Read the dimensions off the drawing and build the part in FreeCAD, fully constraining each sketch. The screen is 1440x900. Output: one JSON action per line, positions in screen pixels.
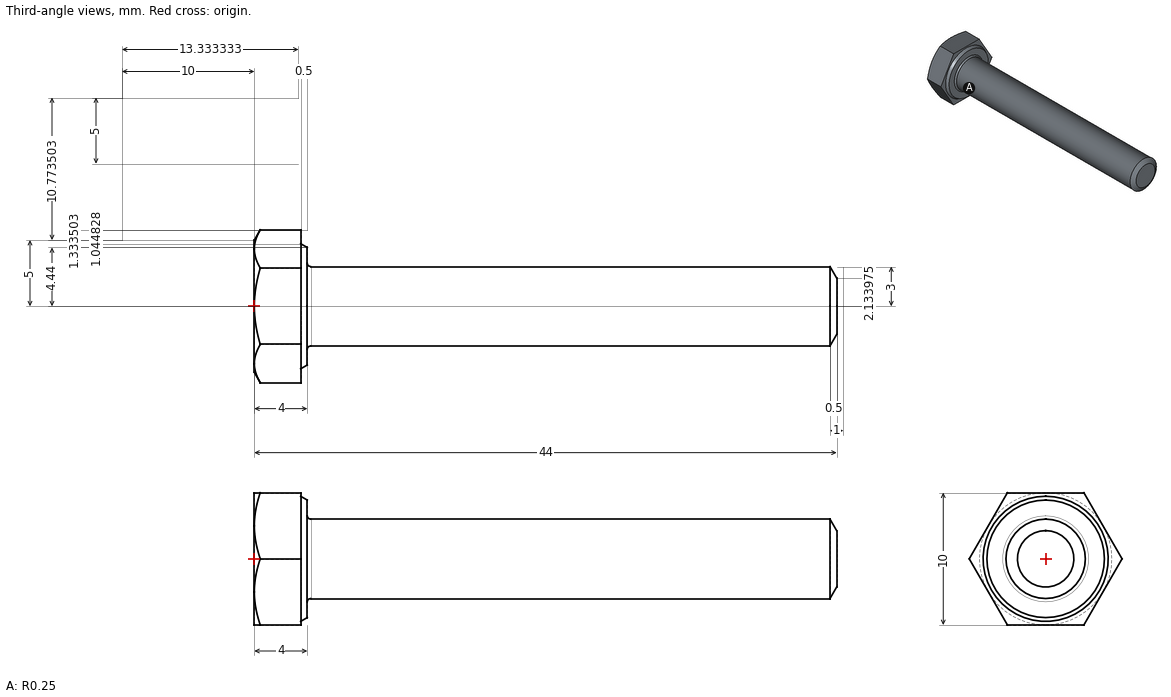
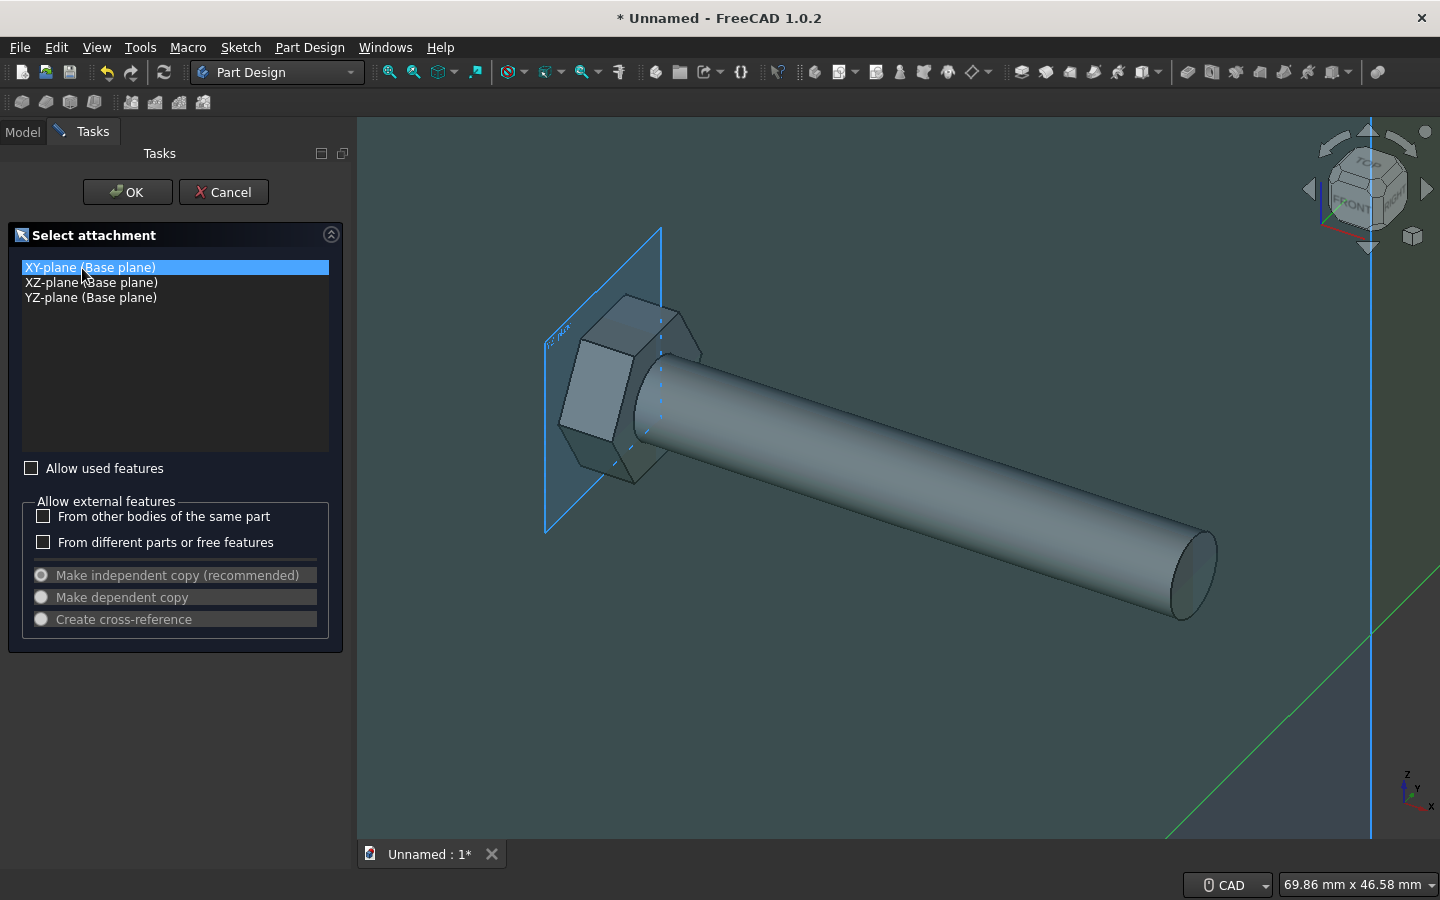
{"action": "left_click", "coordinate": [128, 192]}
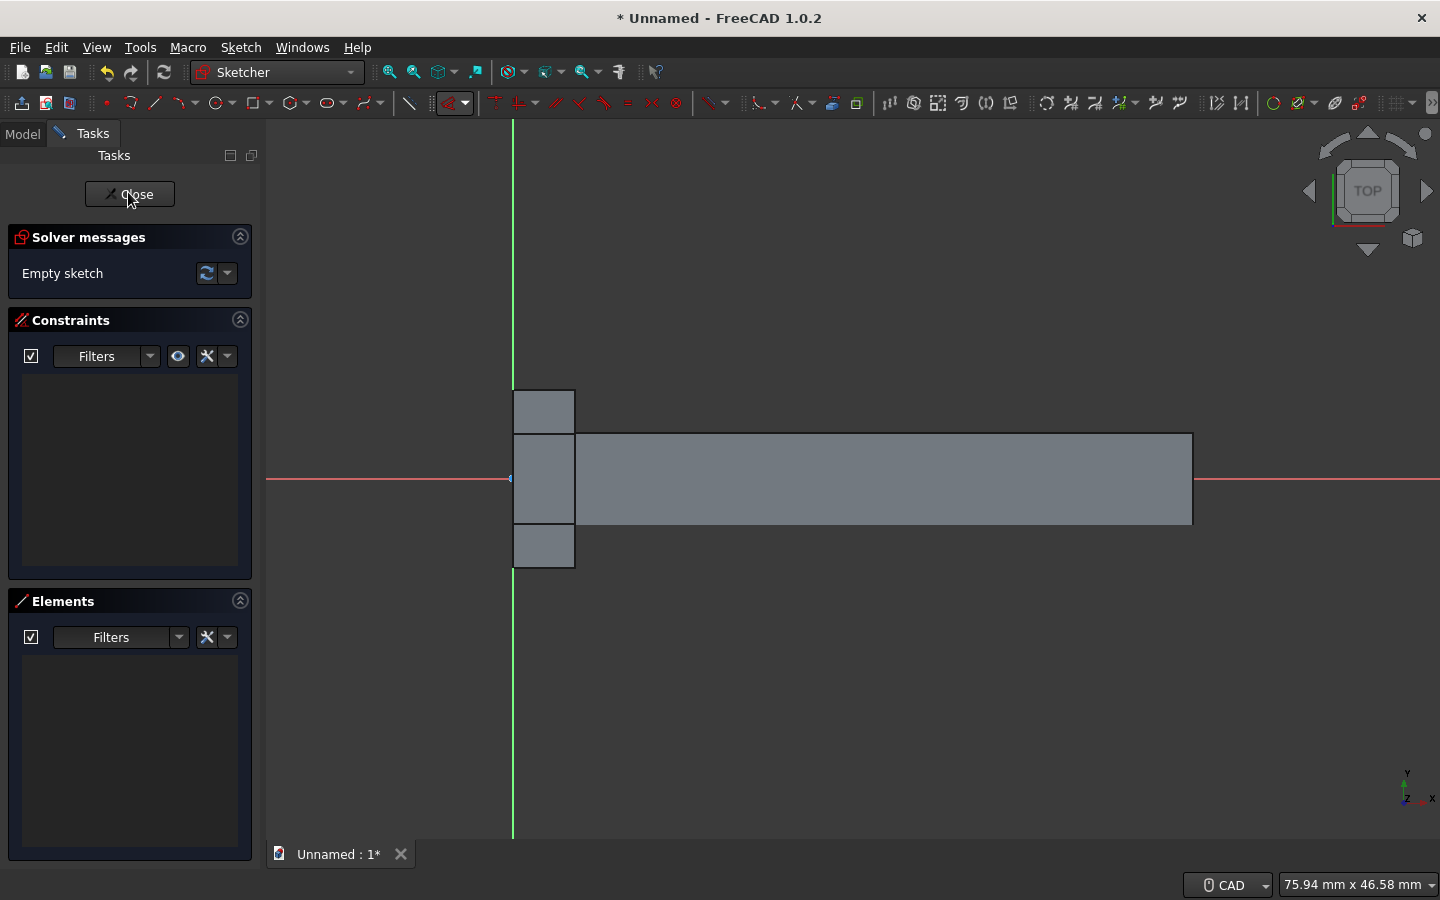
{"action": "left_click", "coordinate": [70, 104]}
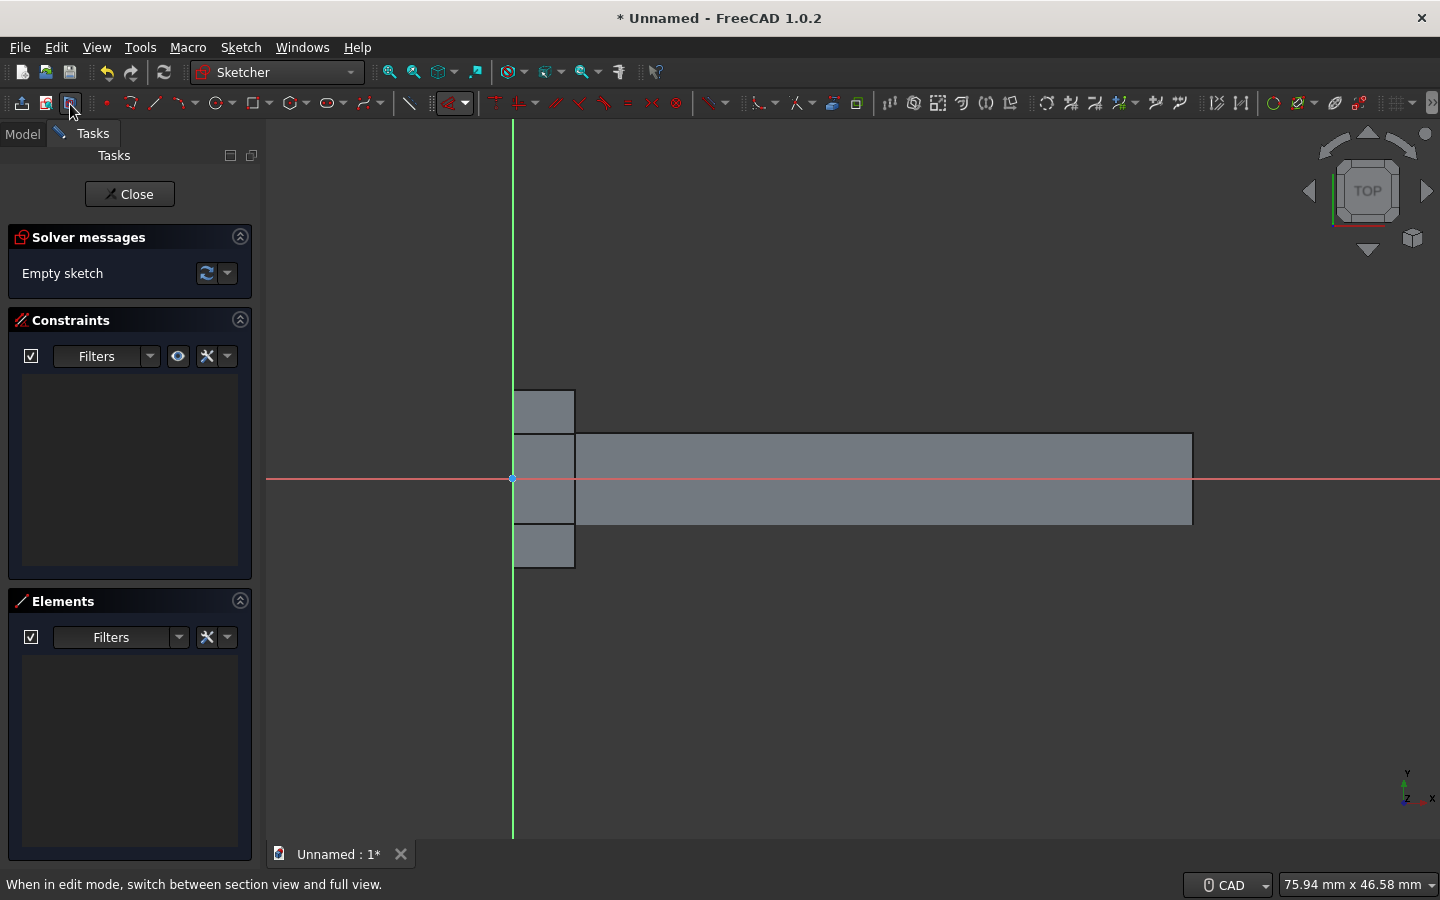
{"action": "scroll", "coordinate": [294, 209], "scroll_direction": "up", "scroll_amount": 3}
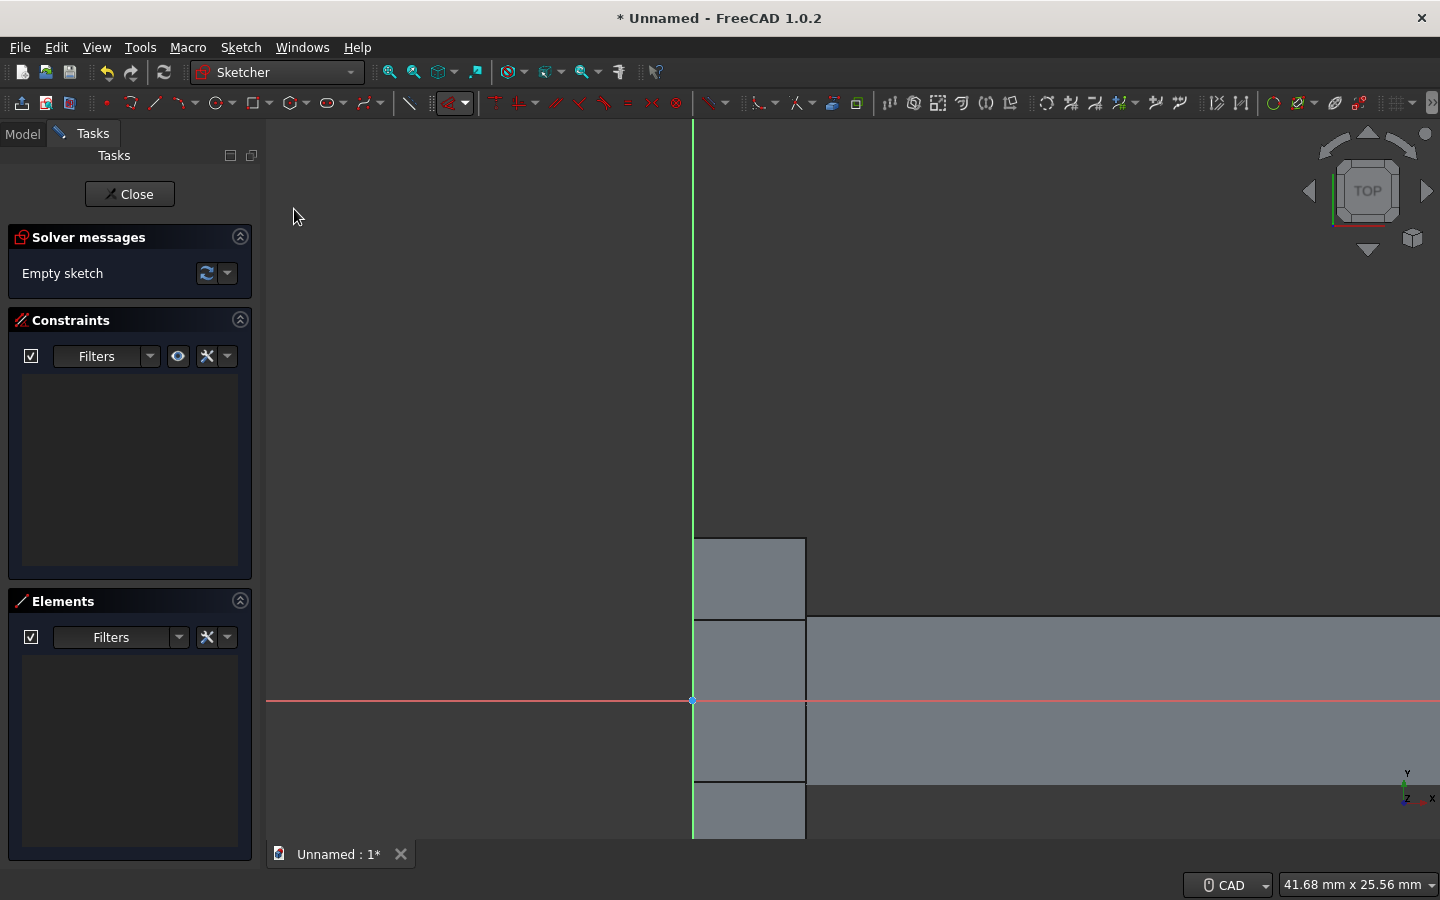
{"action": "left_click", "coordinate": [132, 104]}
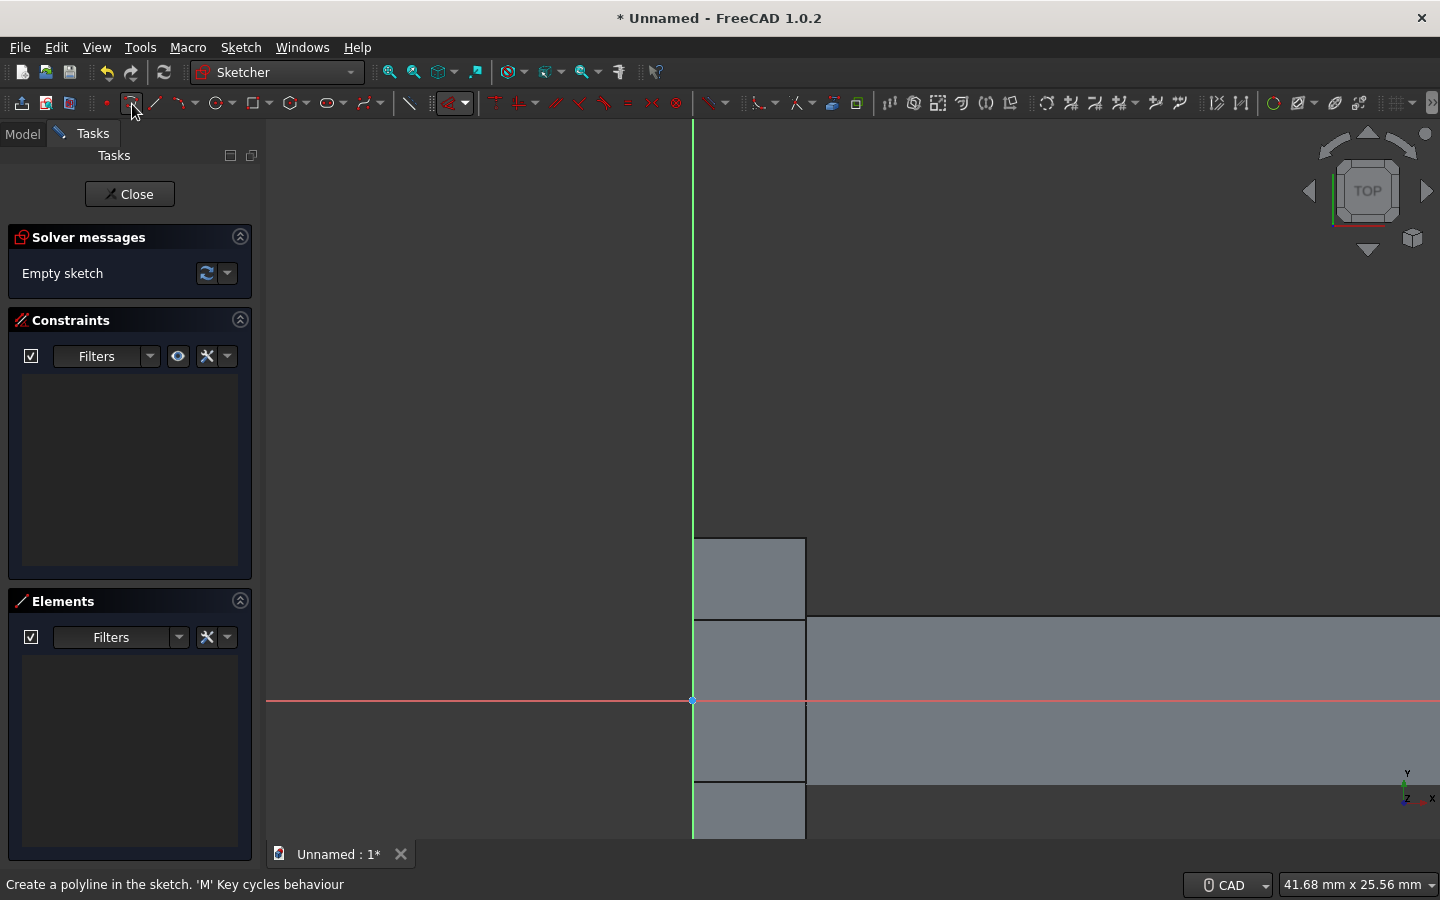
{"action": "left_click", "coordinate": [693, 560]}
{"action": "left_click", "coordinate": [787, 397]}
{"action": "left_click", "coordinate": [787, 257]}
{"action": "left_click", "coordinate": [411, 257]}
{"action": "left_click", "coordinate": [411, 560]}
{"action": "left_click", "coordinate": [693, 561]}
{"action": "key", "text": "Escape"}
{"action": "key", "text": "Escape"}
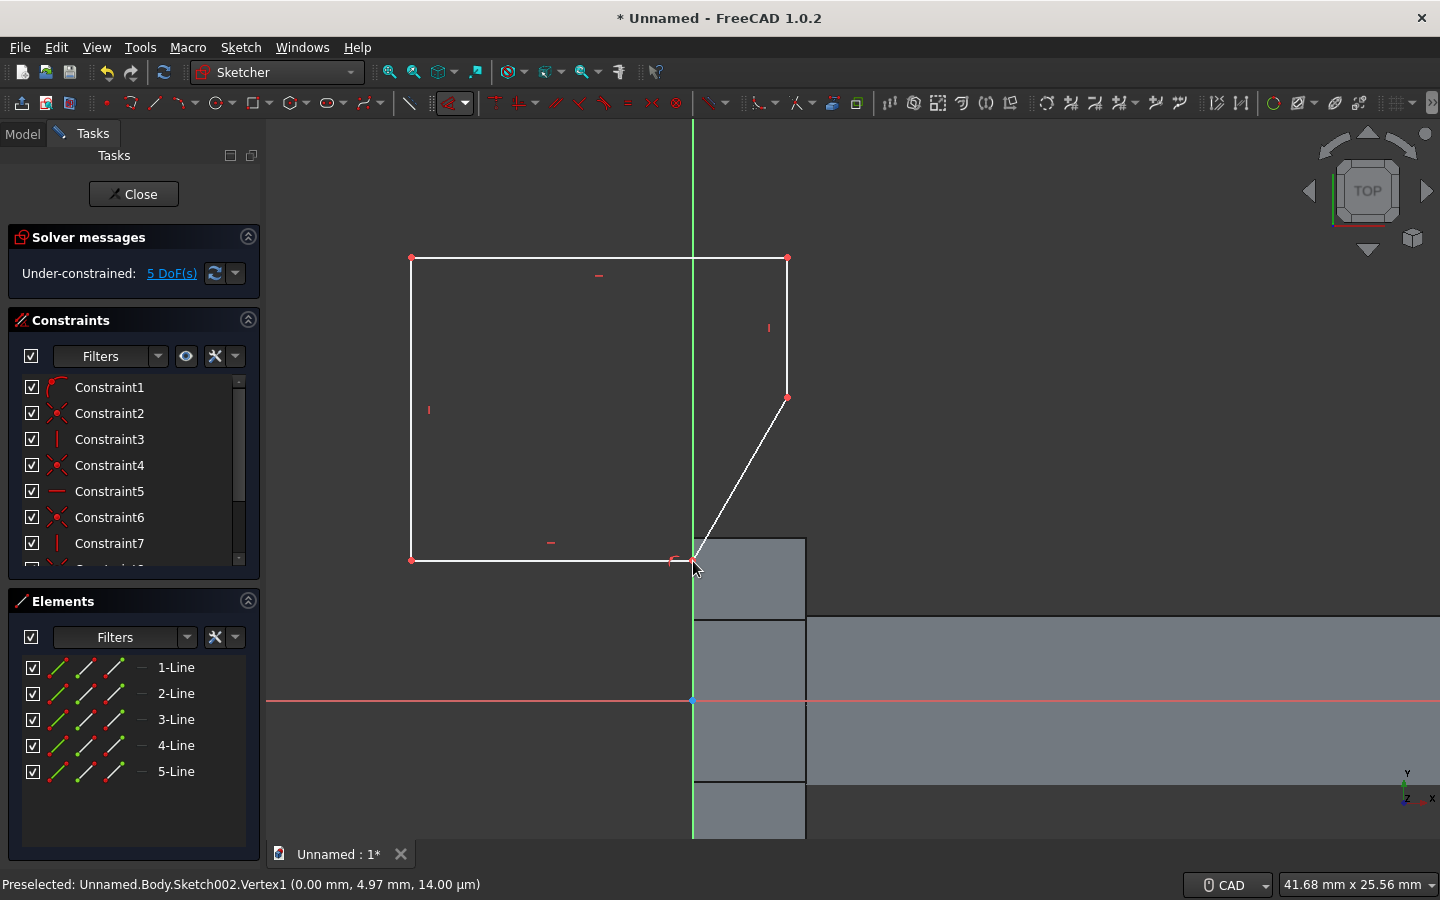
{"action": "left_click", "coordinate": [787, 356]}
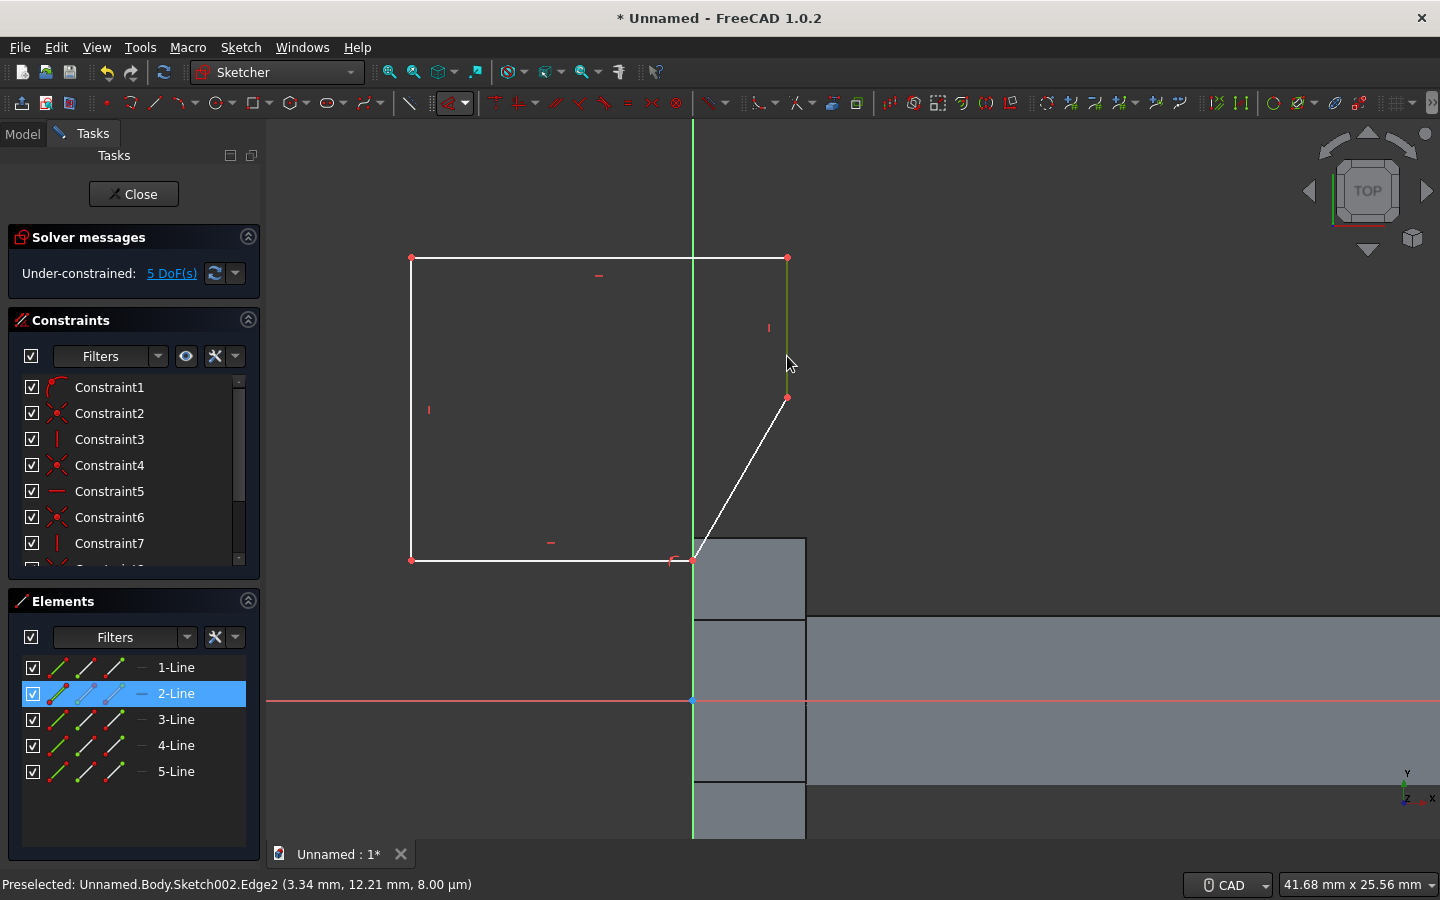
{"action": "left_click", "coordinate": [468, 104]}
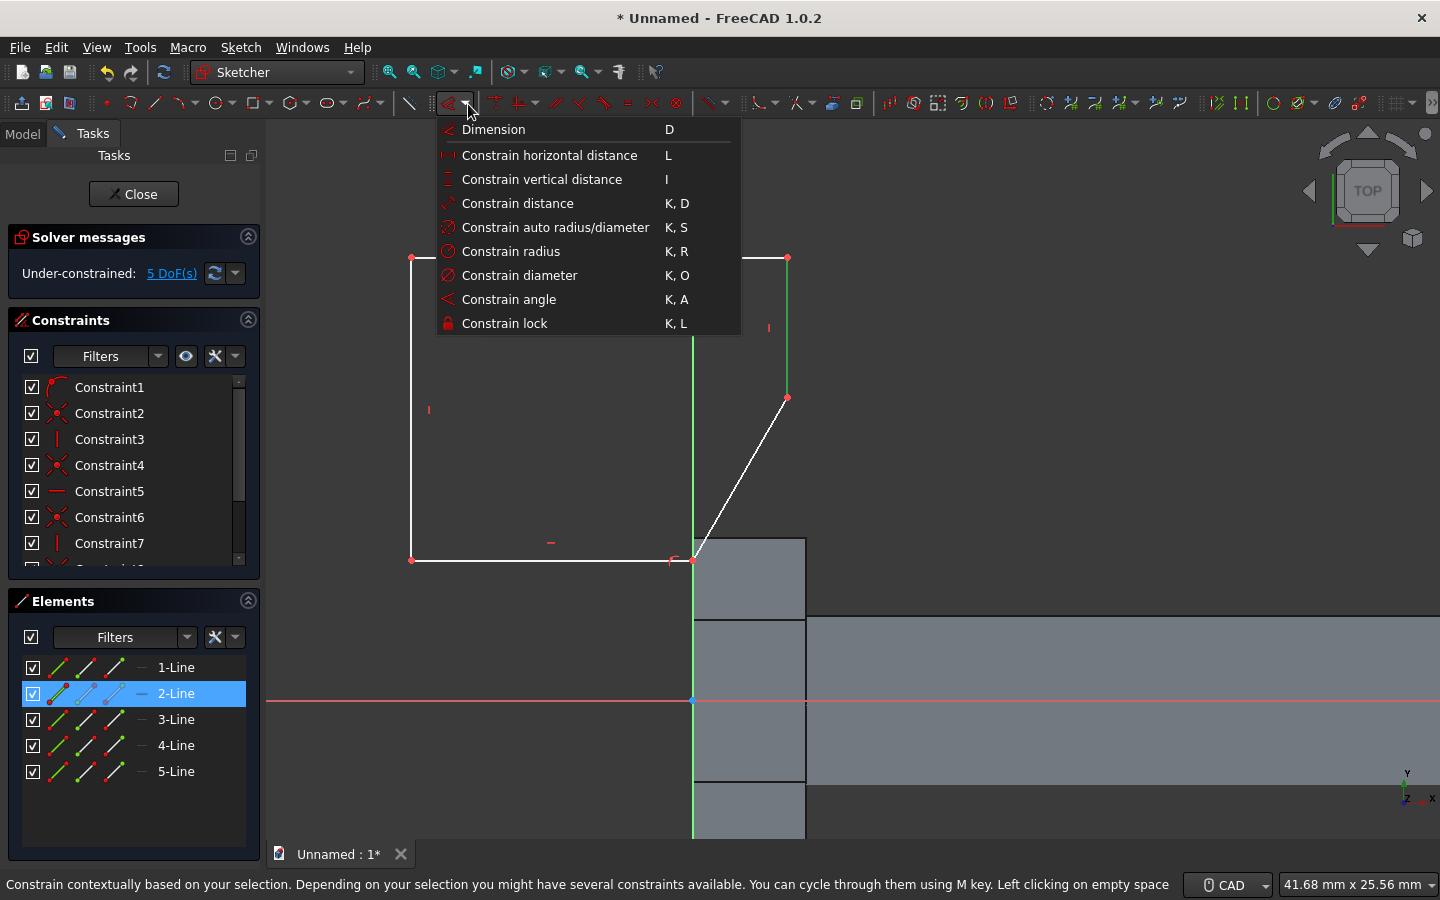
{"action": "left_click", "coordinate": [589, 179]}